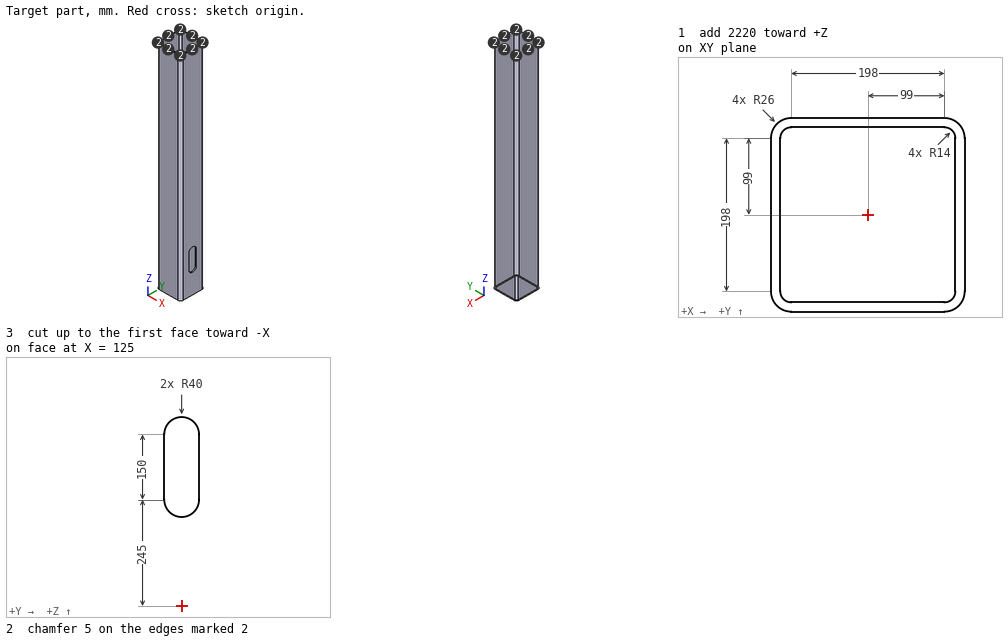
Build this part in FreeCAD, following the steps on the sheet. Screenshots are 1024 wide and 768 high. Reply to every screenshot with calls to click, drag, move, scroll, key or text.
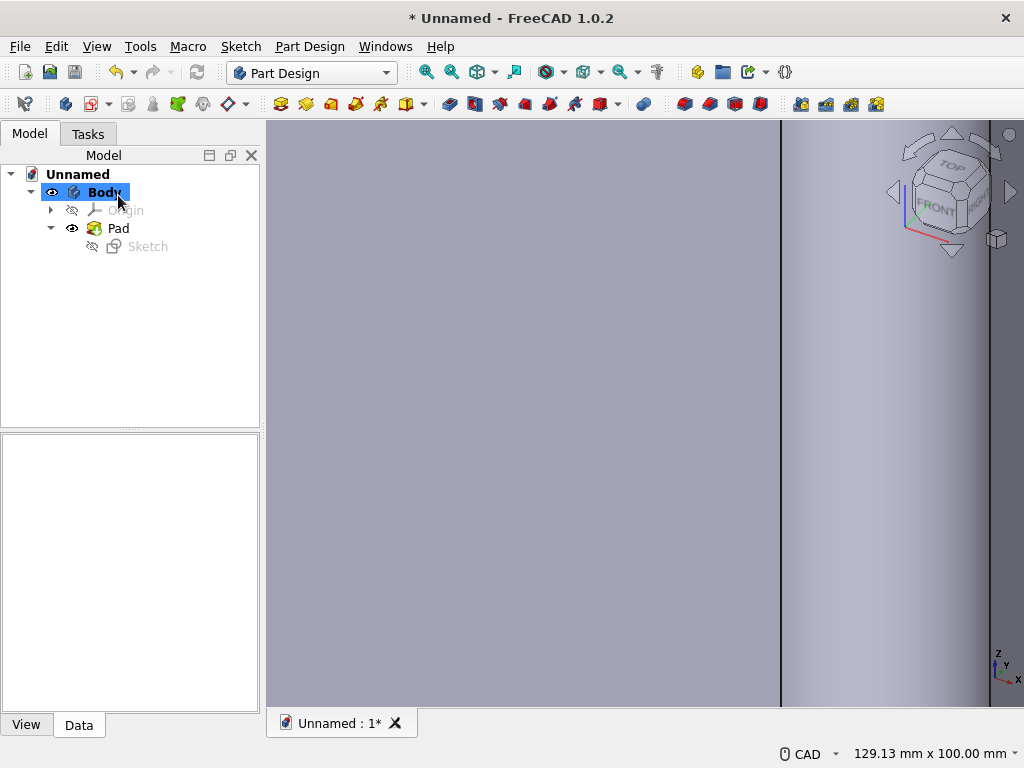
click(427, 72)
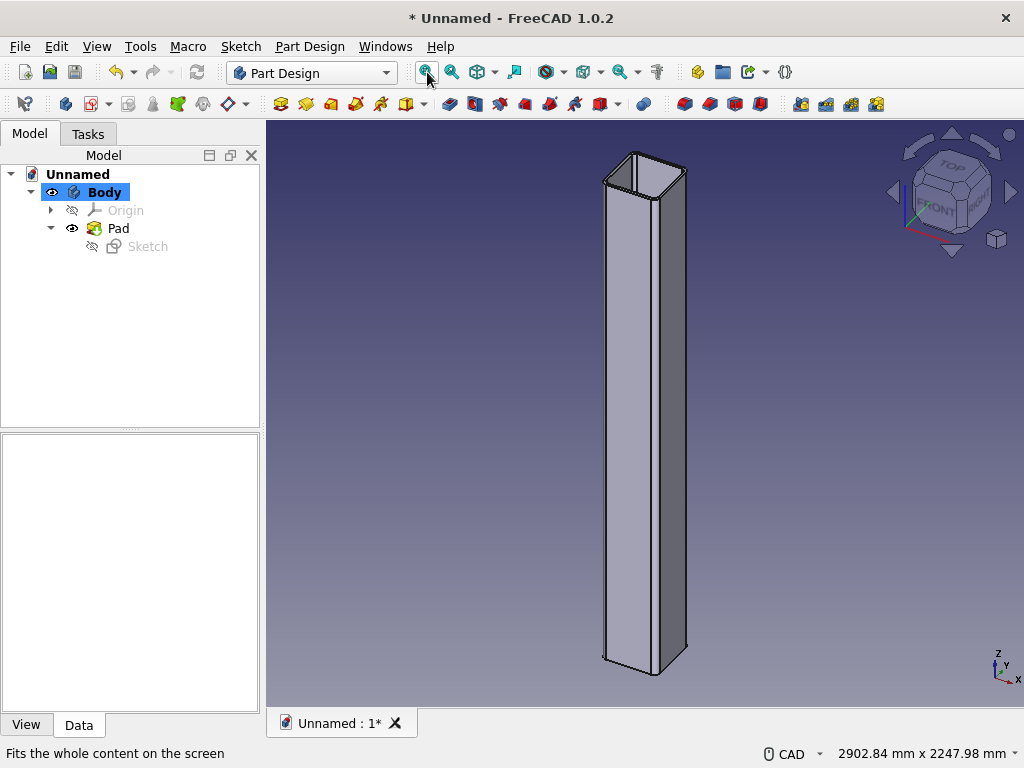
click(629, 191)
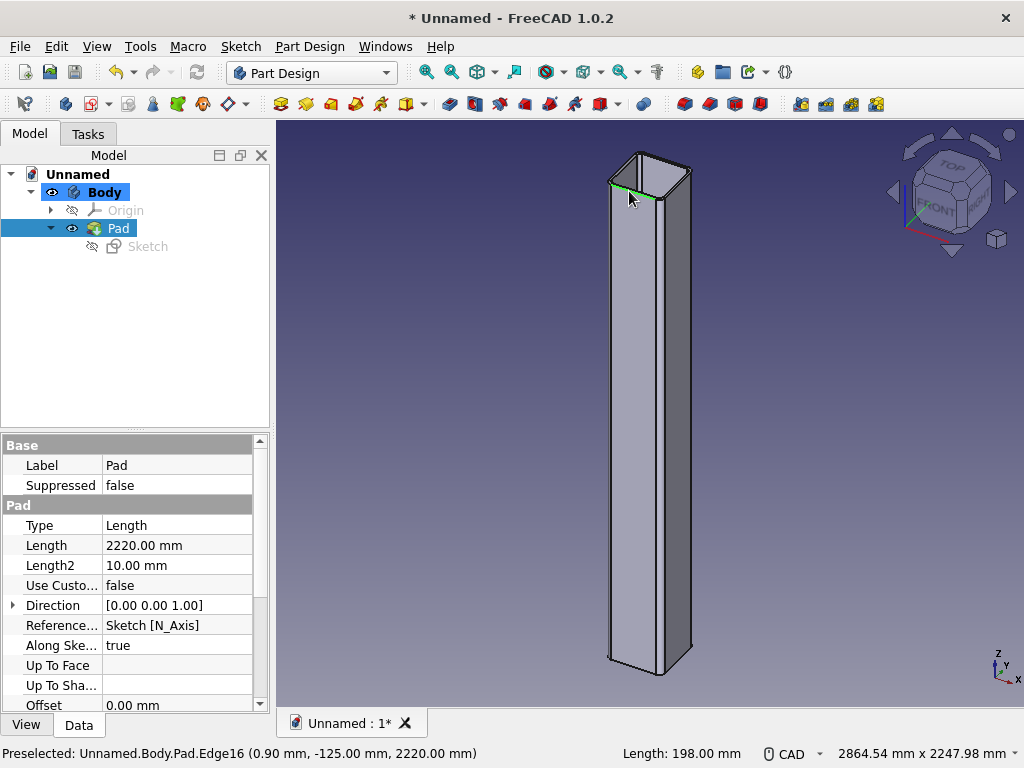
click(661, 199, ctrl)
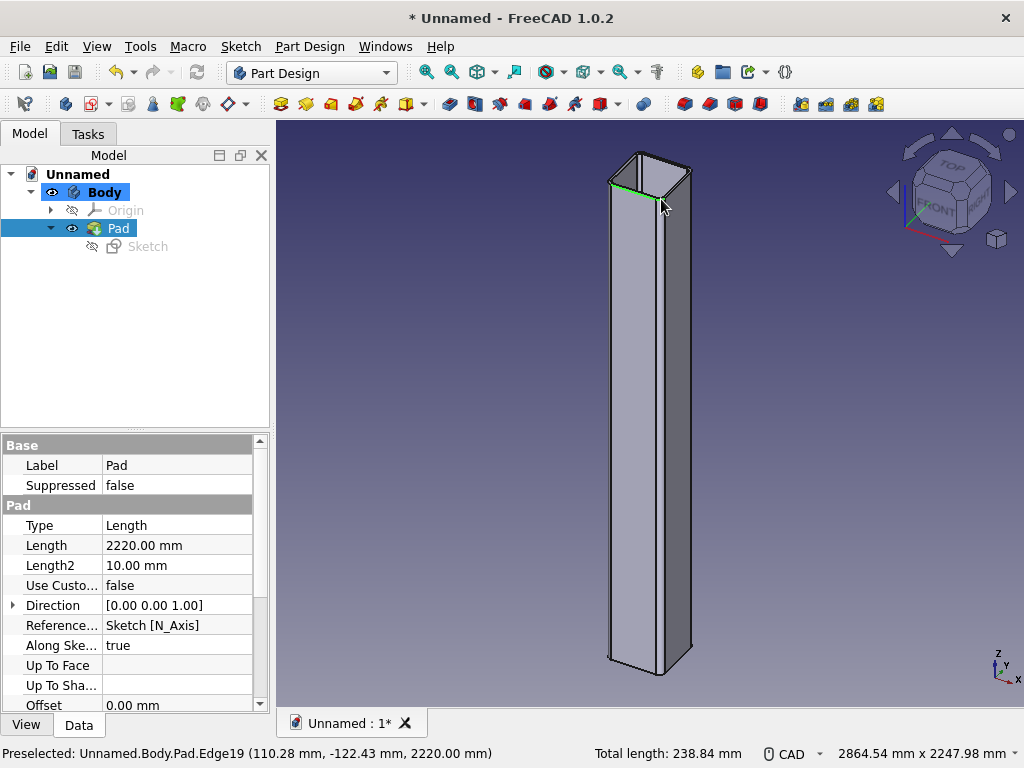
click(678, 184, ctrl)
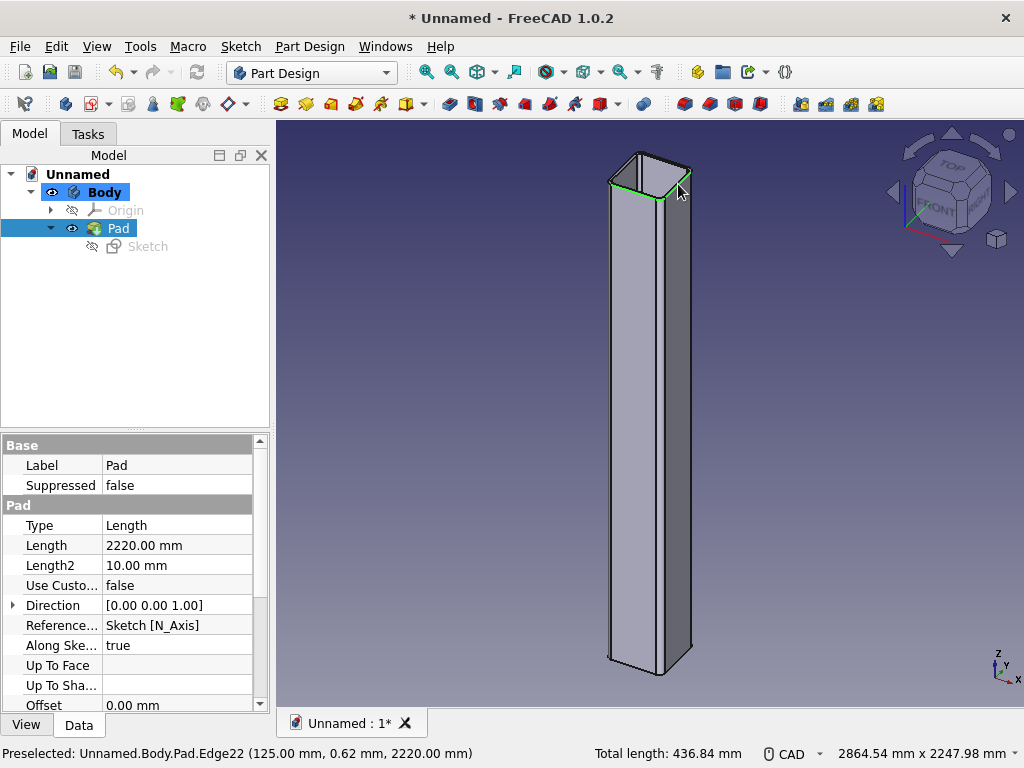
scroll(608, 182, up, 7)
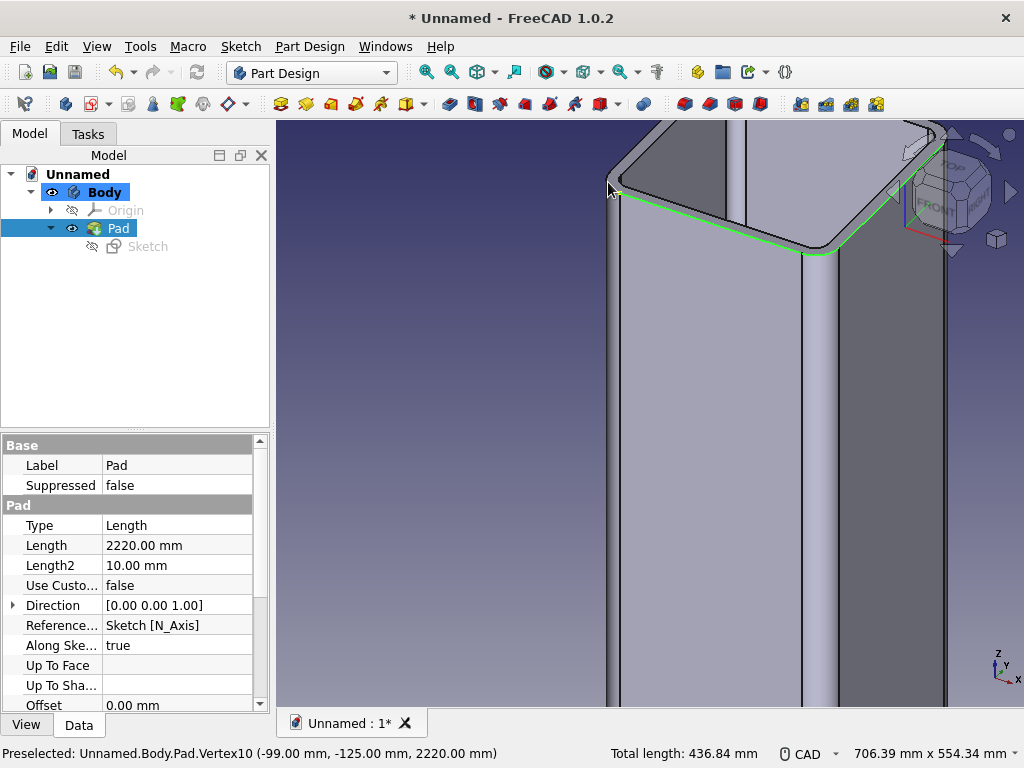
click(607, 183, ctrl)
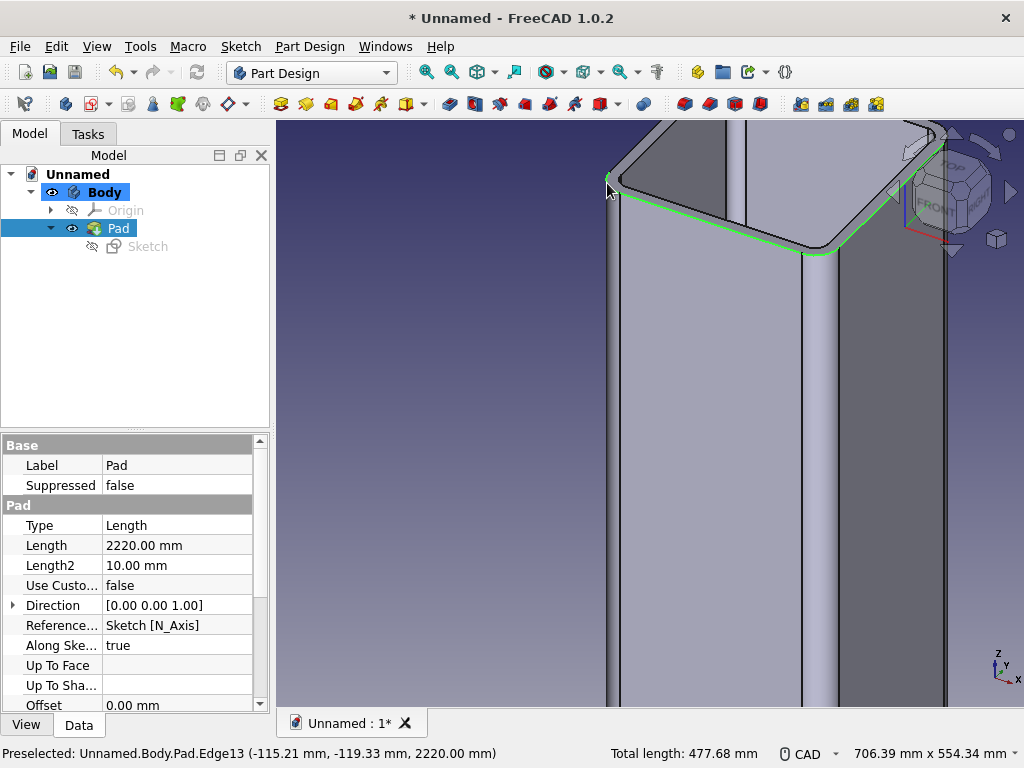
click(427, 72)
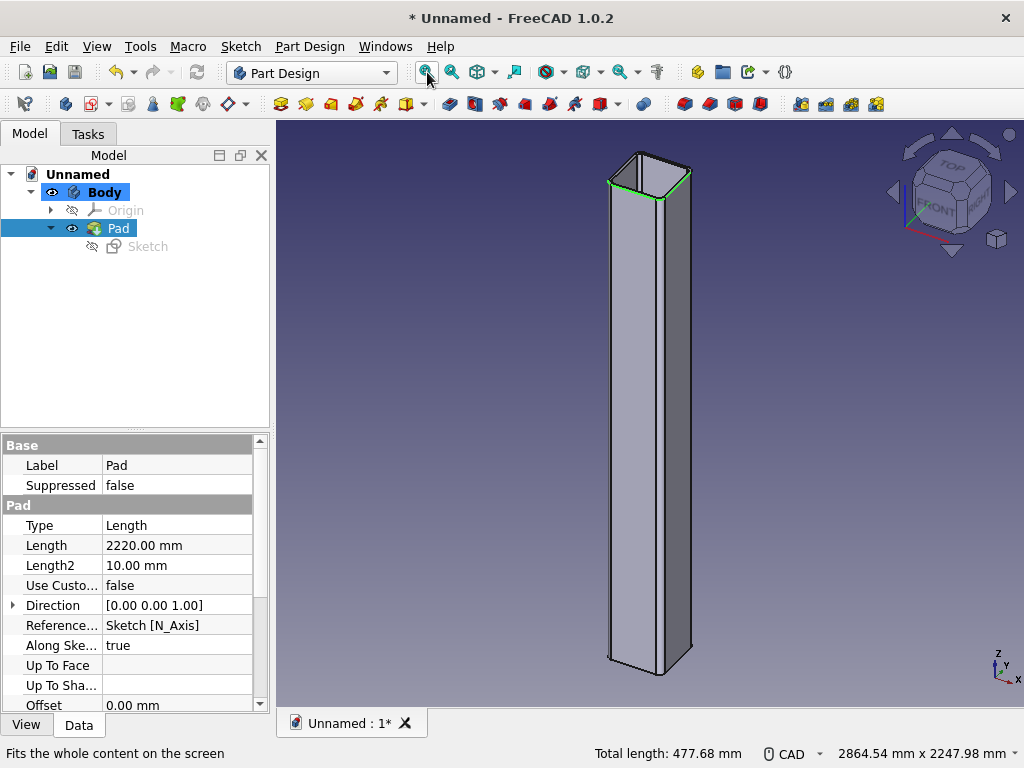
key(0)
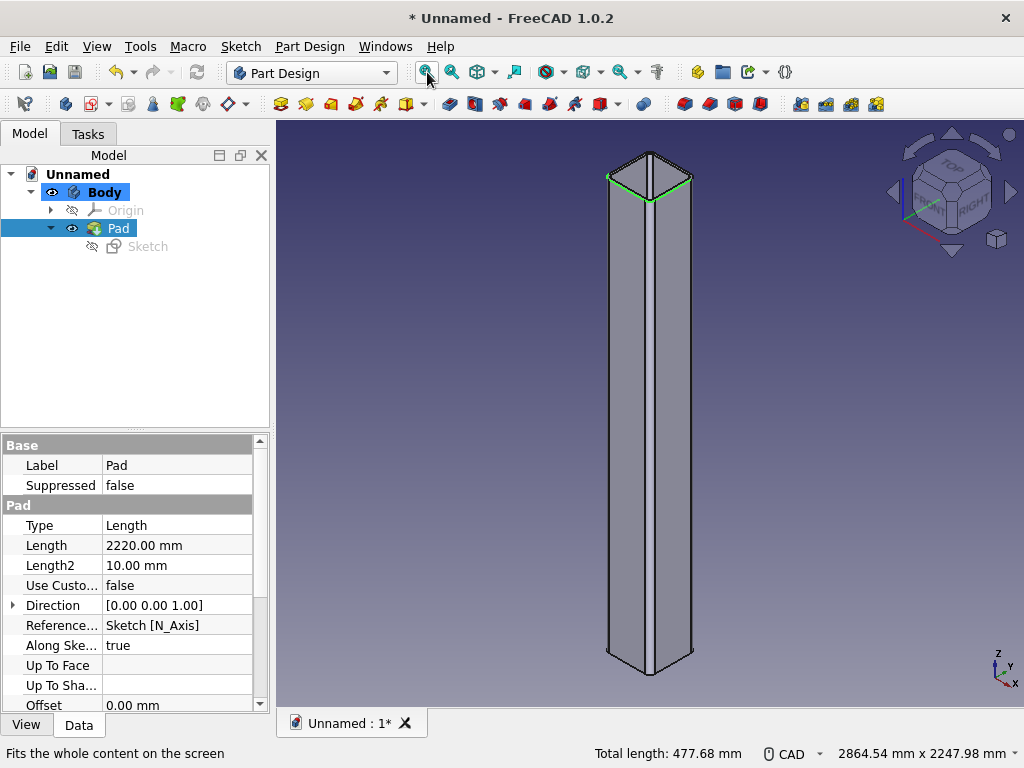
scroll(693, 176, up, 7)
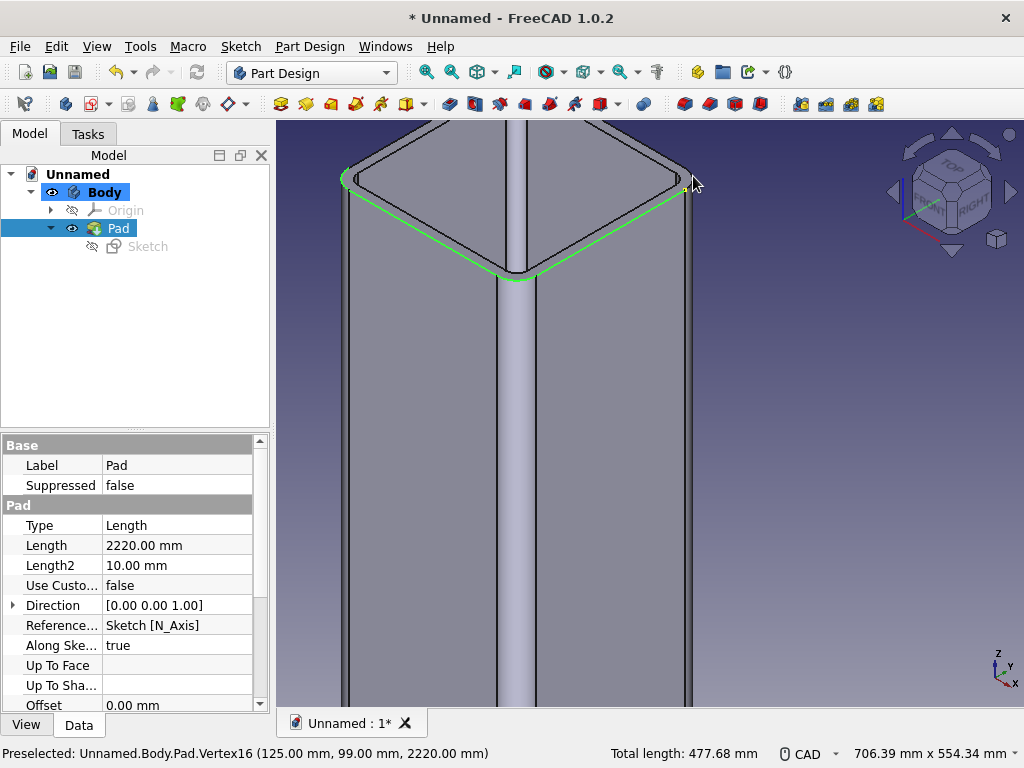
click(693, 178, ctrl)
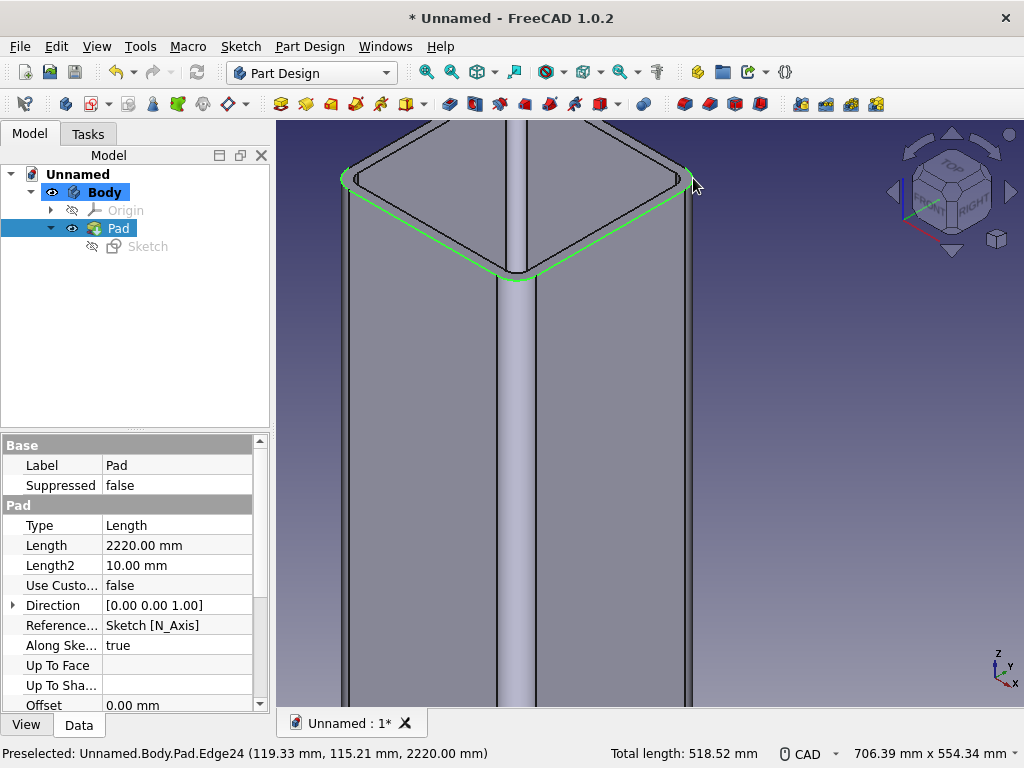
click(427, 72)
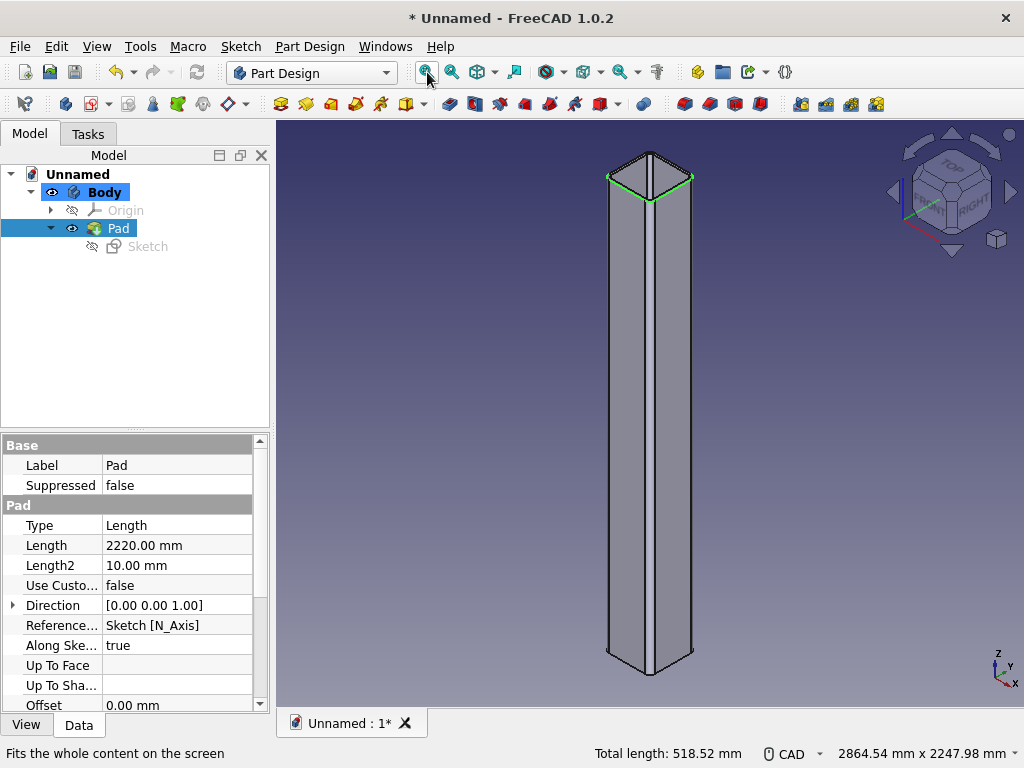
key(2)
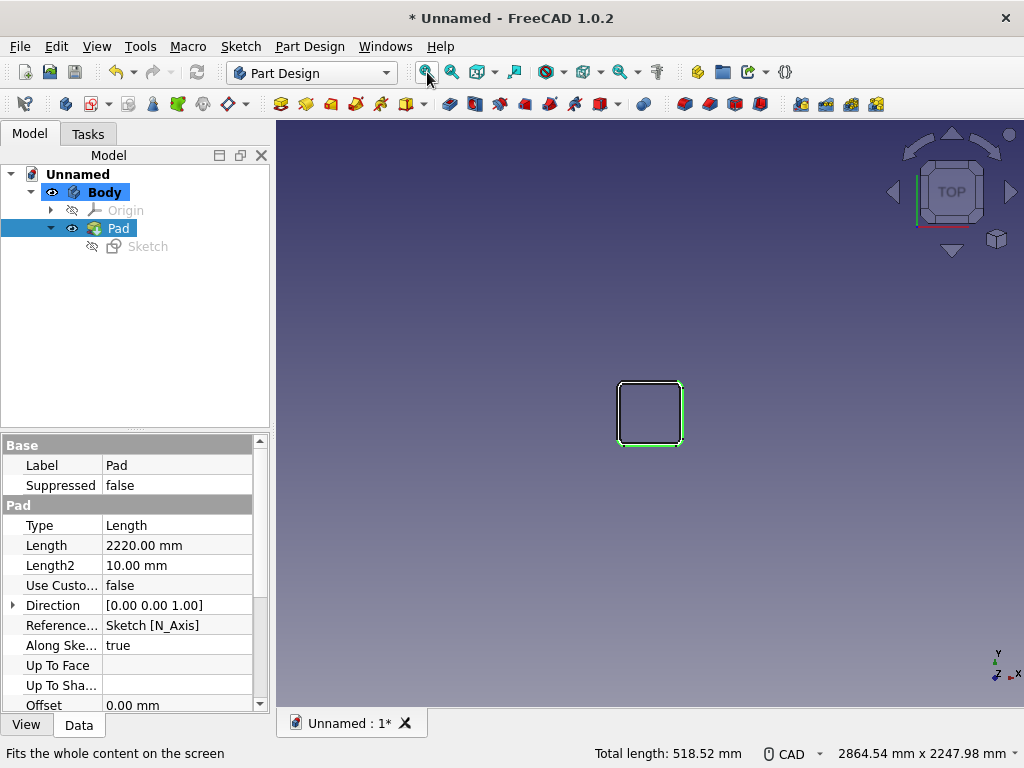
click(427, 72)